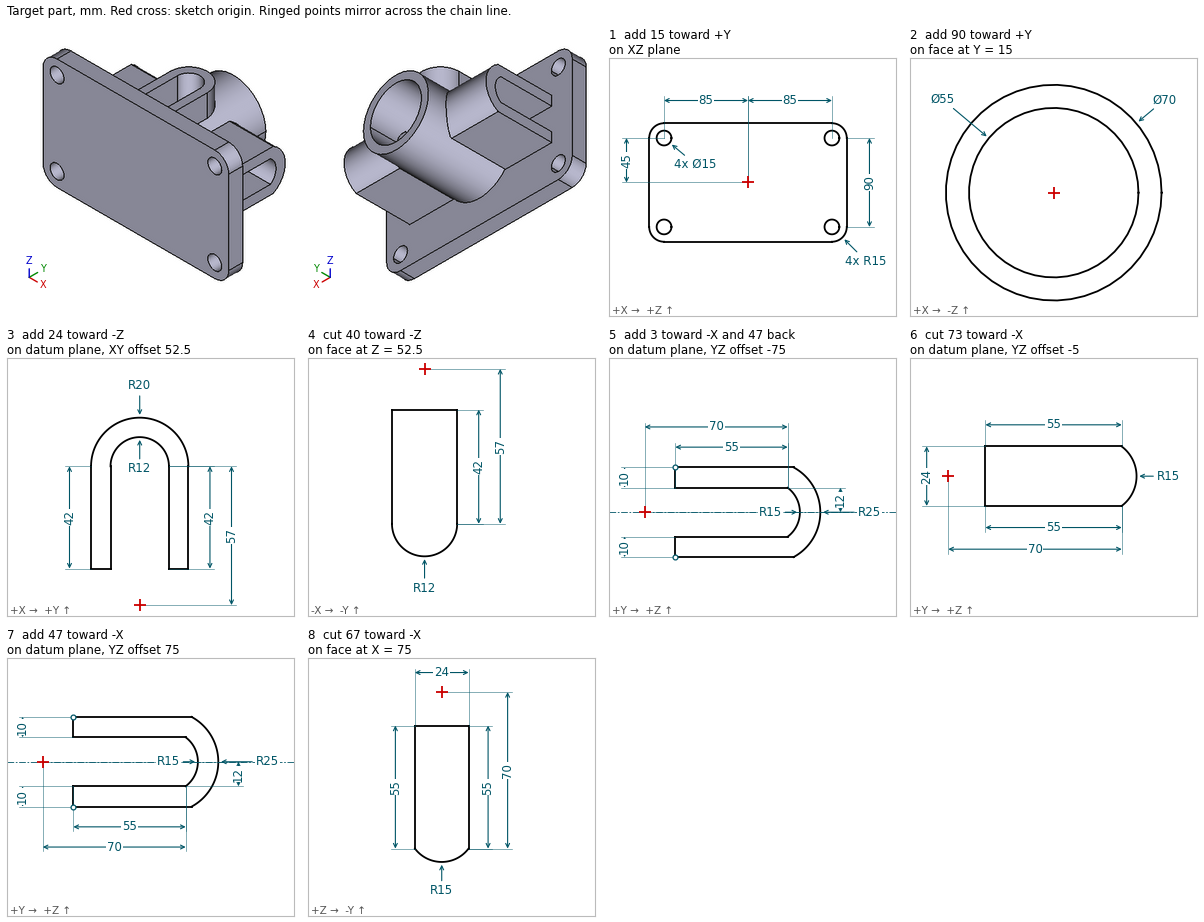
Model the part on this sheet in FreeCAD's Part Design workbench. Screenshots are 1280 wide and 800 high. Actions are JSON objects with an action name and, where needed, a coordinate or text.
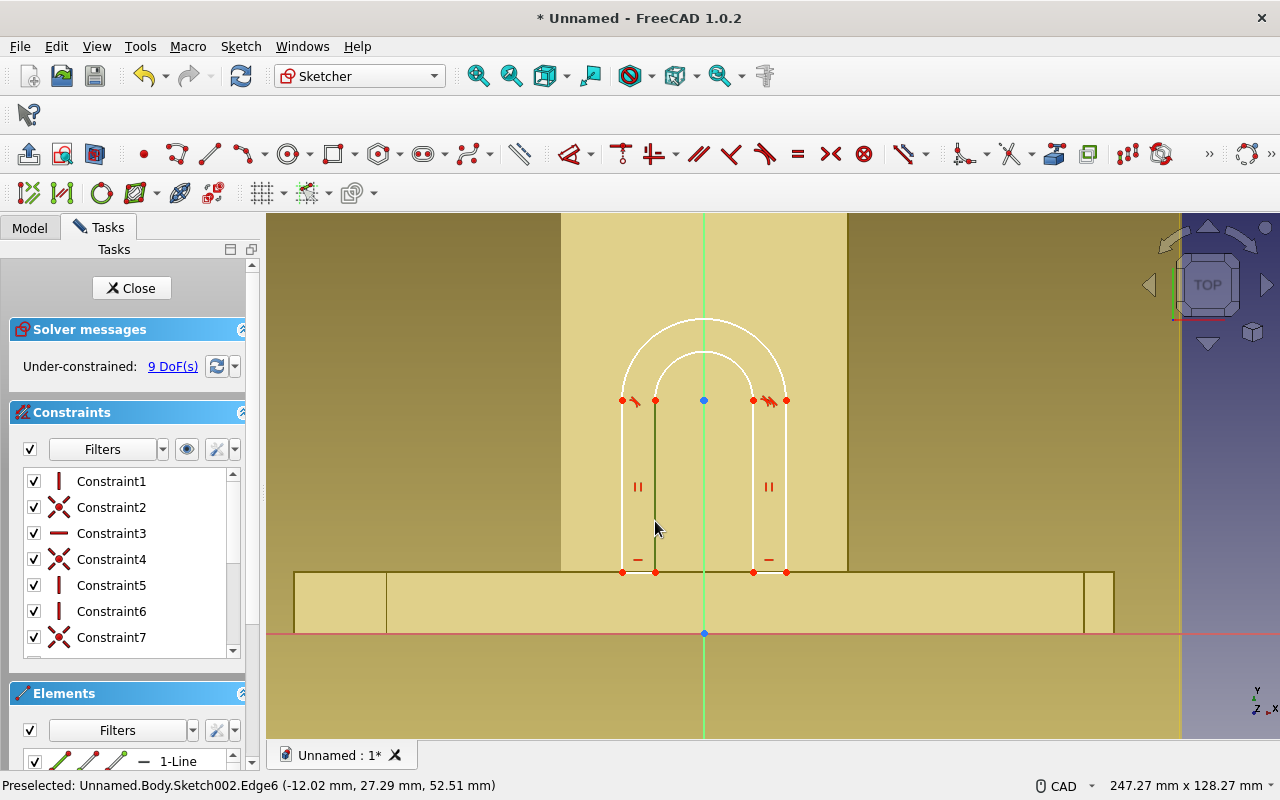
{"action": "left_click", "coordinate": [733, 361]}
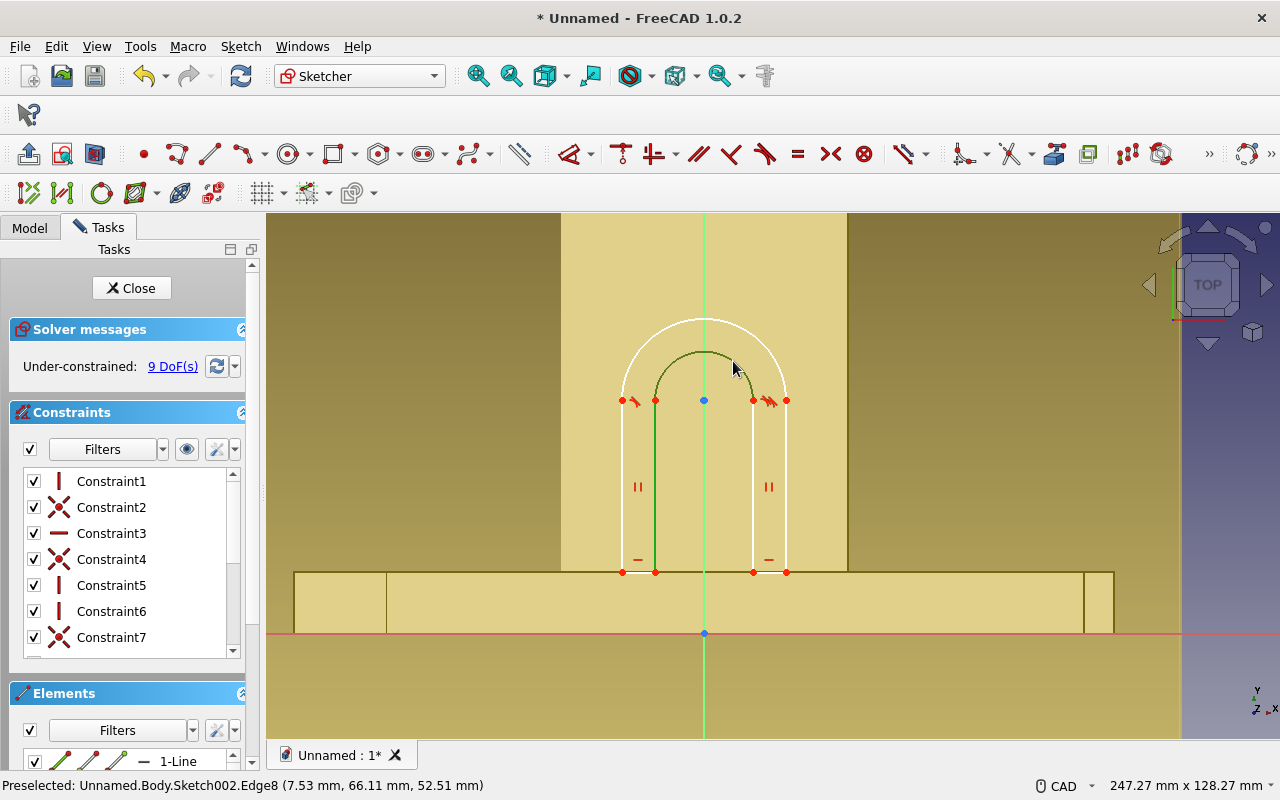
{"action": "key", "text": "t"}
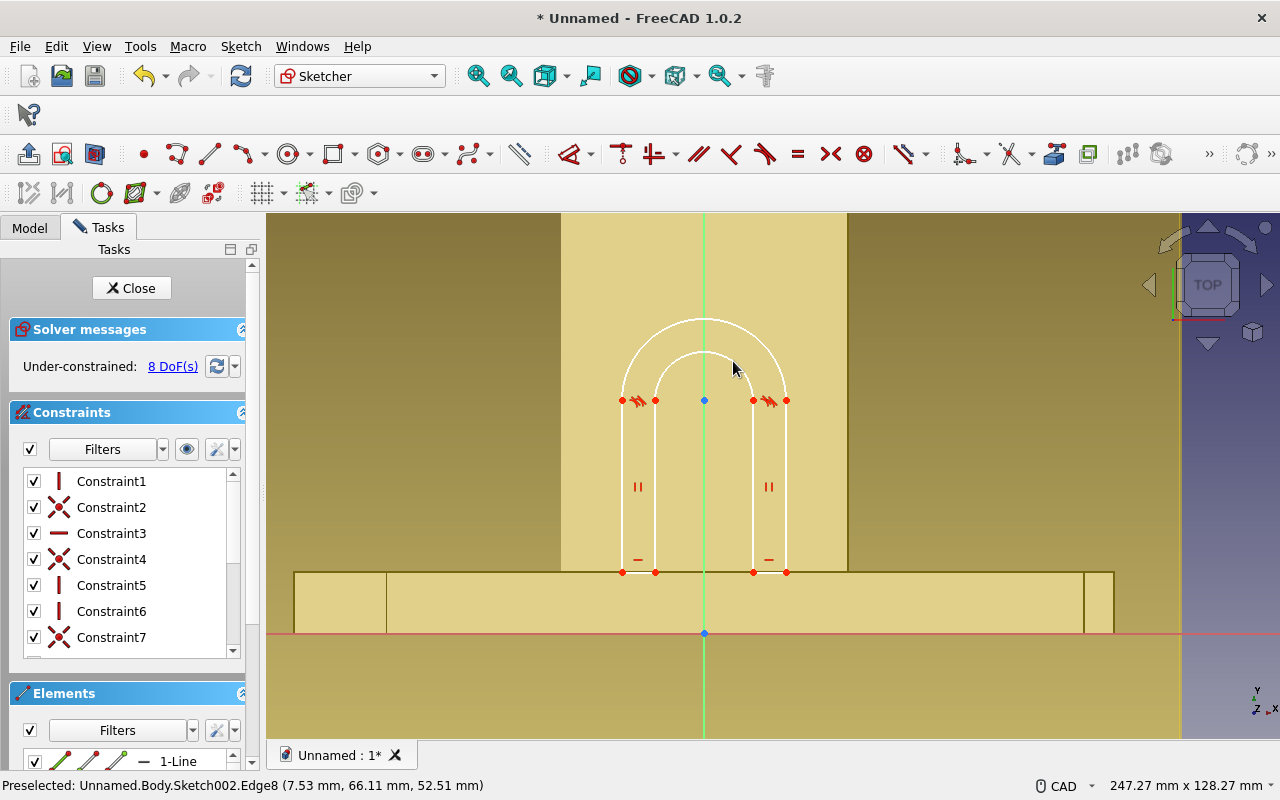
{"action": "left_click", "coordinate": [752, 335]}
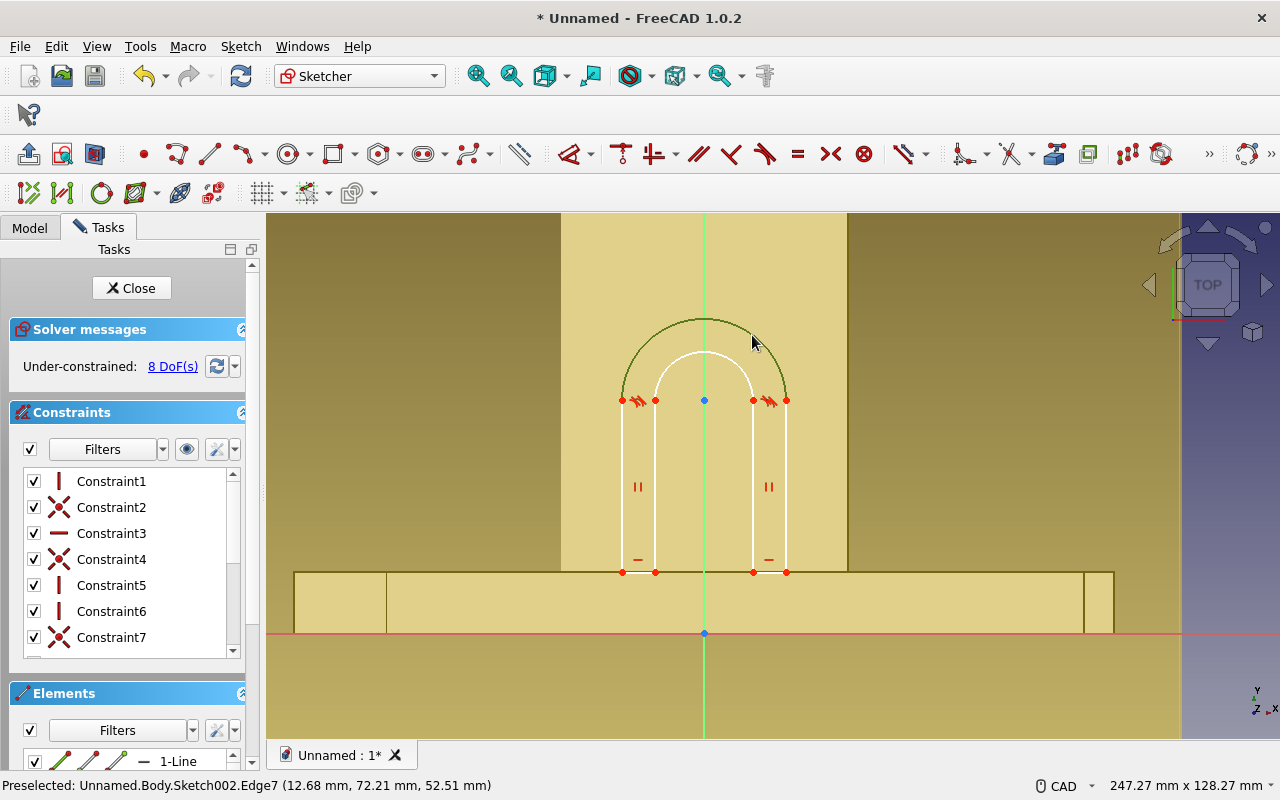
{"action": "left_click", "coordinate": [733, 361]}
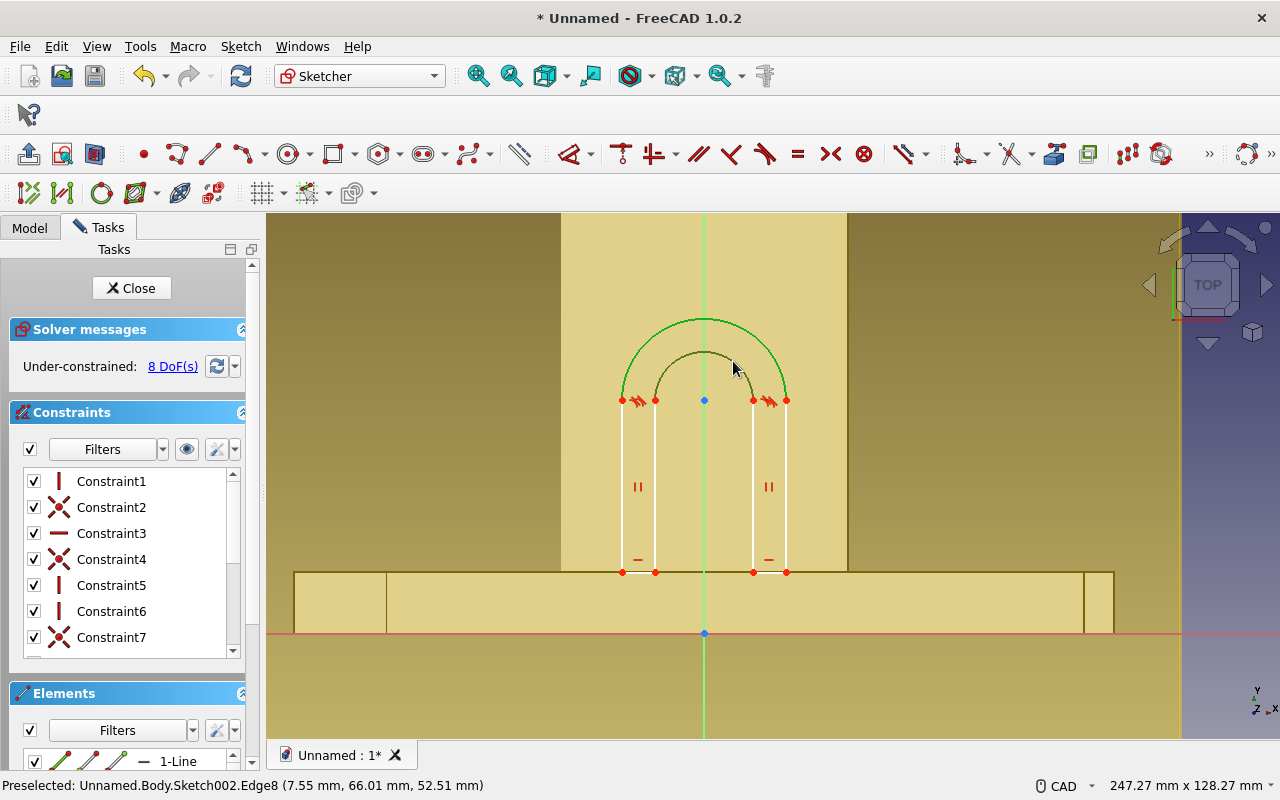
{"action": "left_click", "coordinate": [621, 154]}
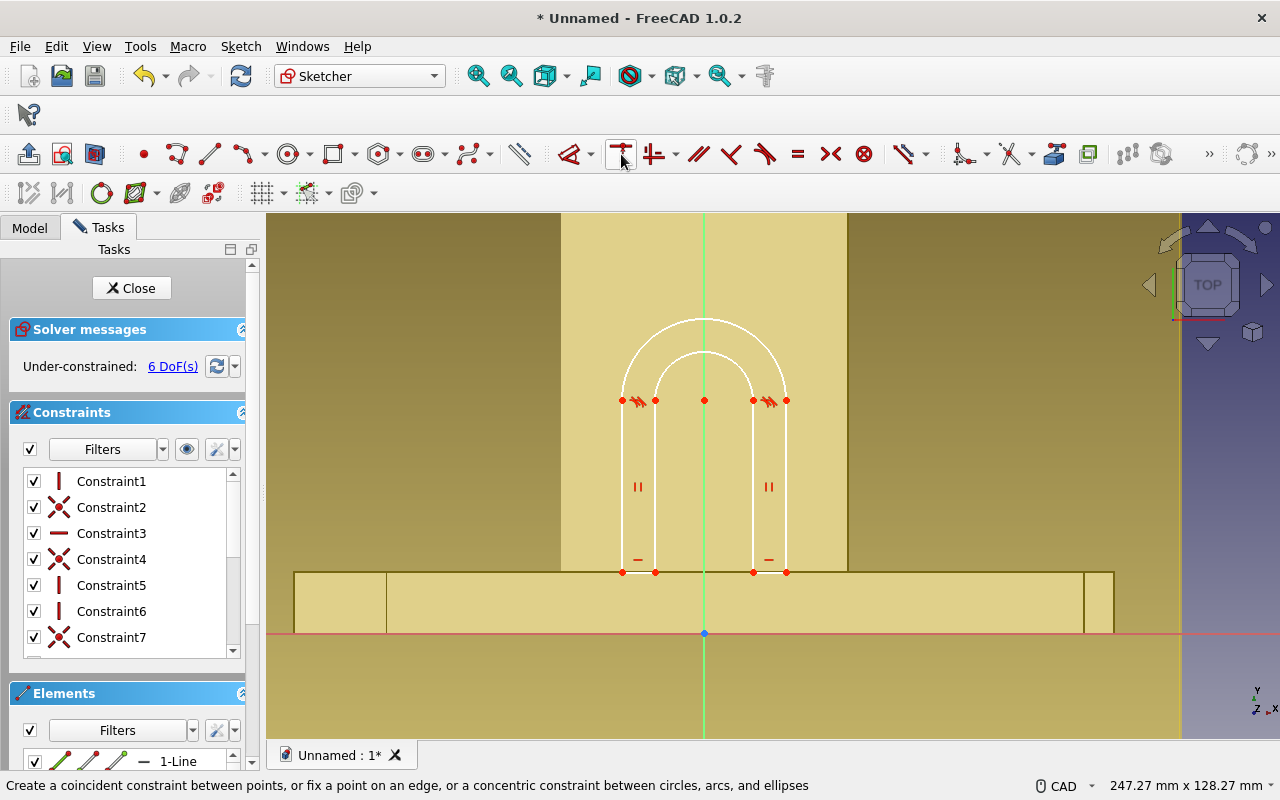
{"action": "left_click", "coordinate": [704, 401]}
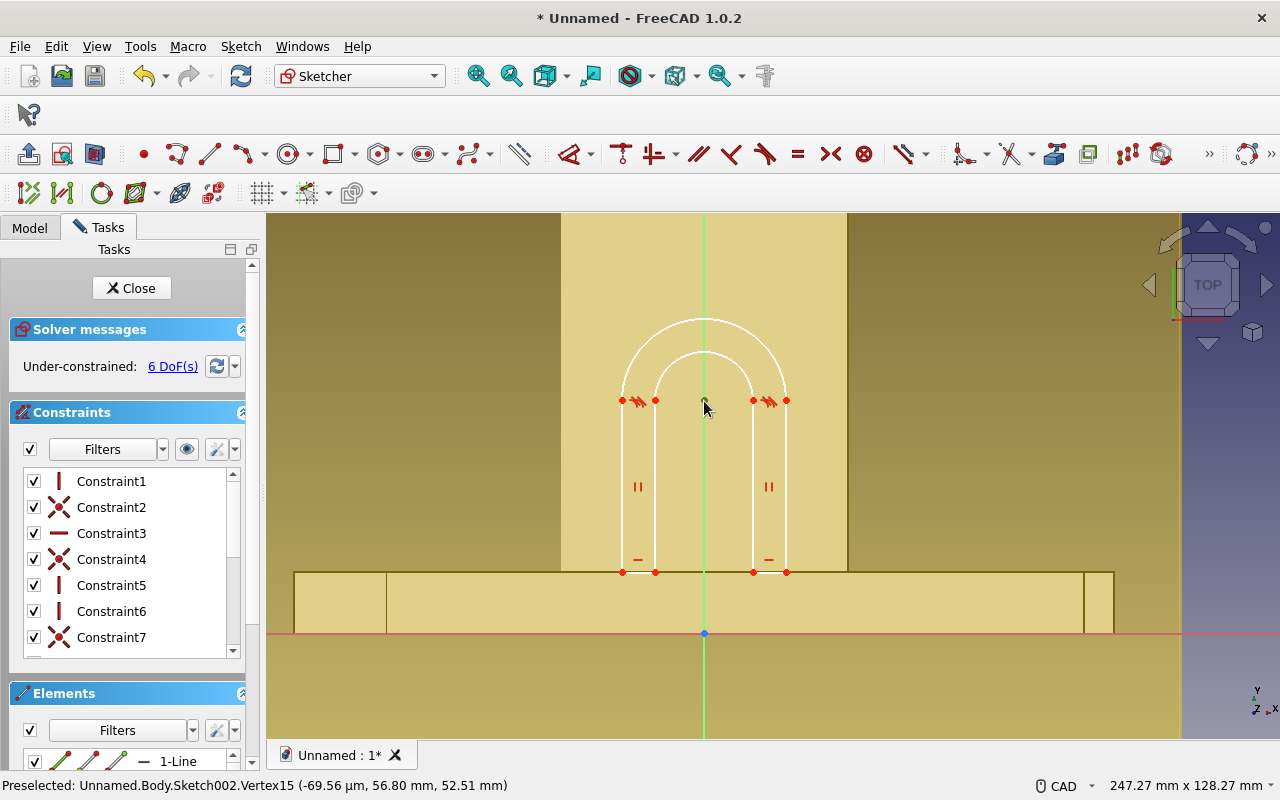
{"action": "left_click", "coordinate": [704, 677]}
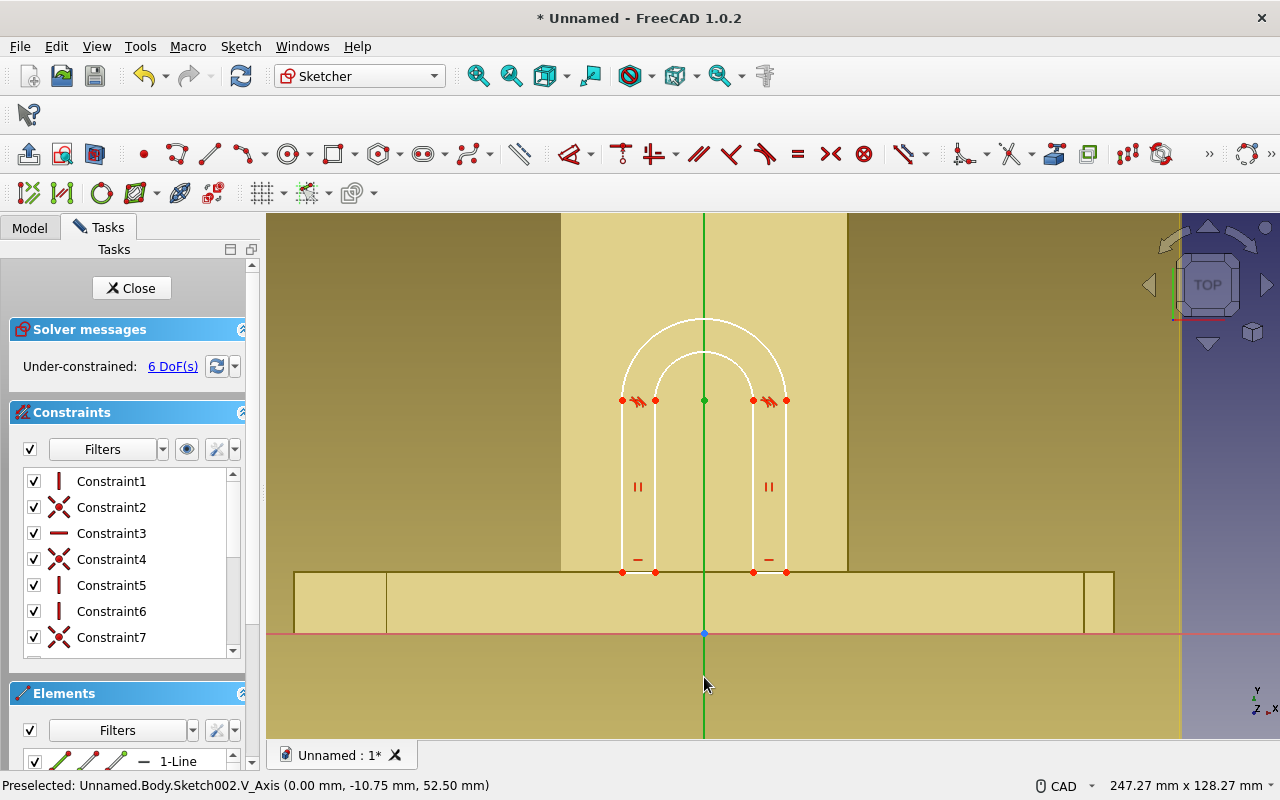
{"action": "key", "text": "c"}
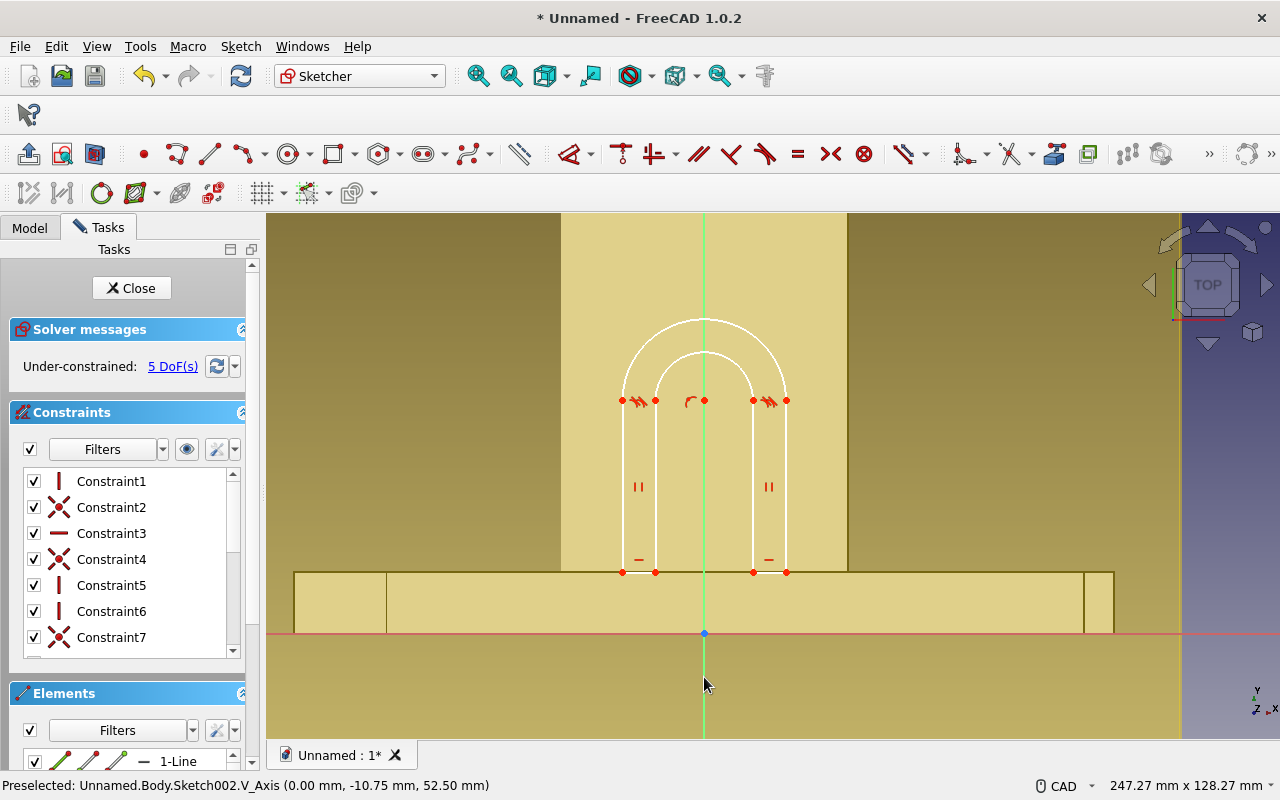
{"action": "left_click", "coordinate": [752, 335]}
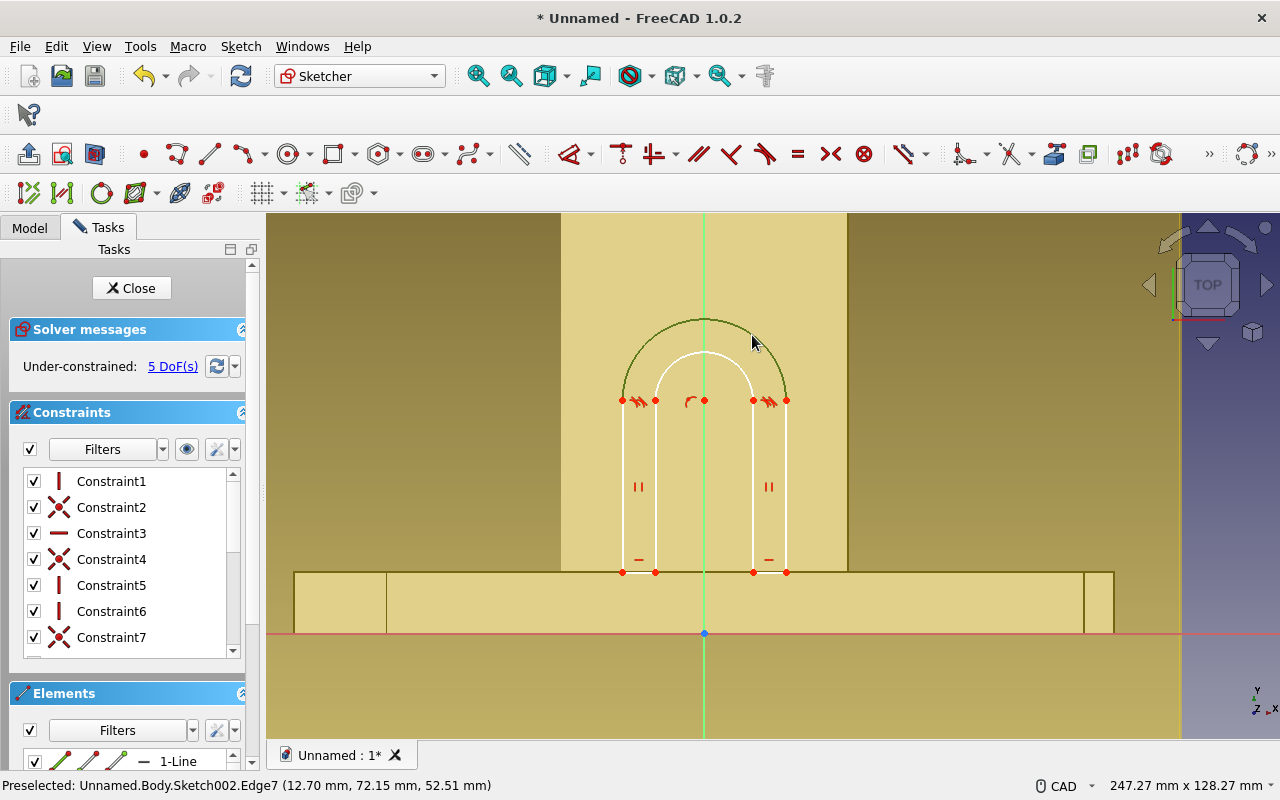
{"action": "key", "text": "k r"}